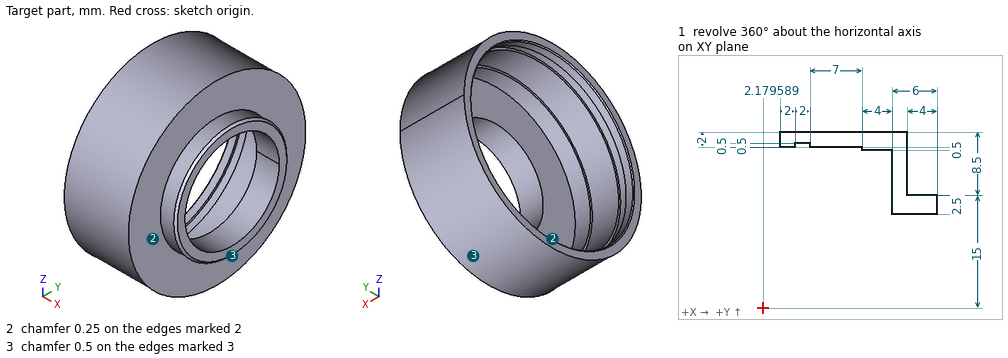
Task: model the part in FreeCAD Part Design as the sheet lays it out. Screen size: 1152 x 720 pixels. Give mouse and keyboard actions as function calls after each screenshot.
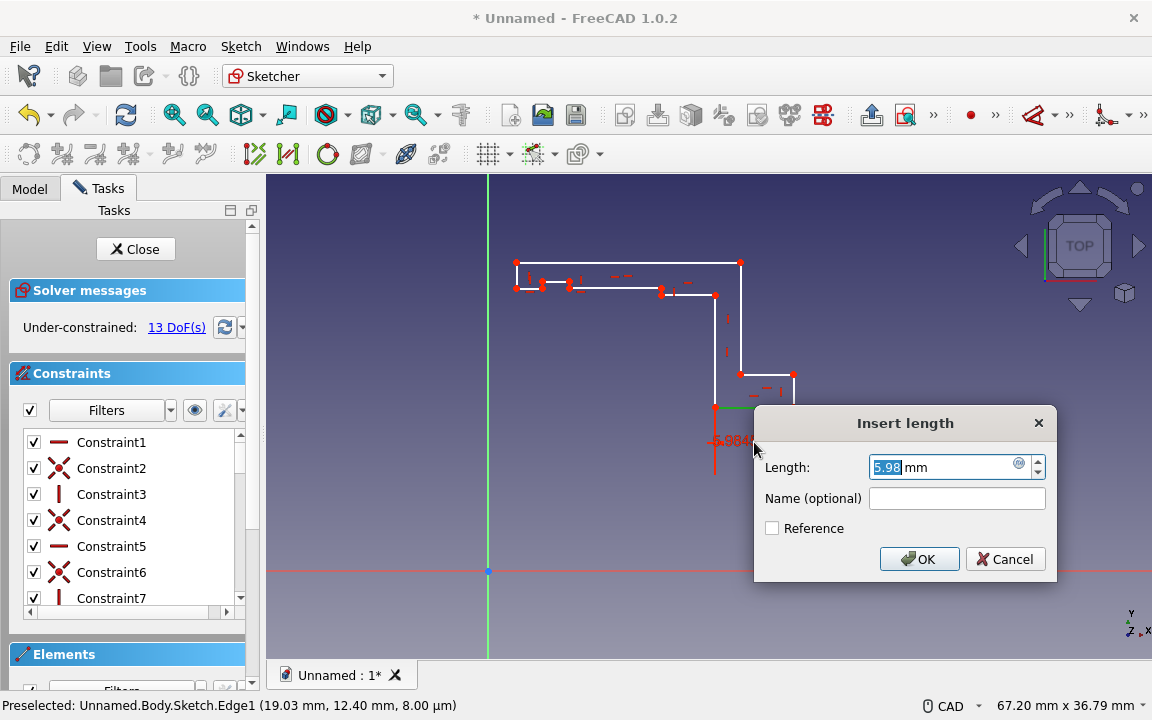
text(6)
key(Return)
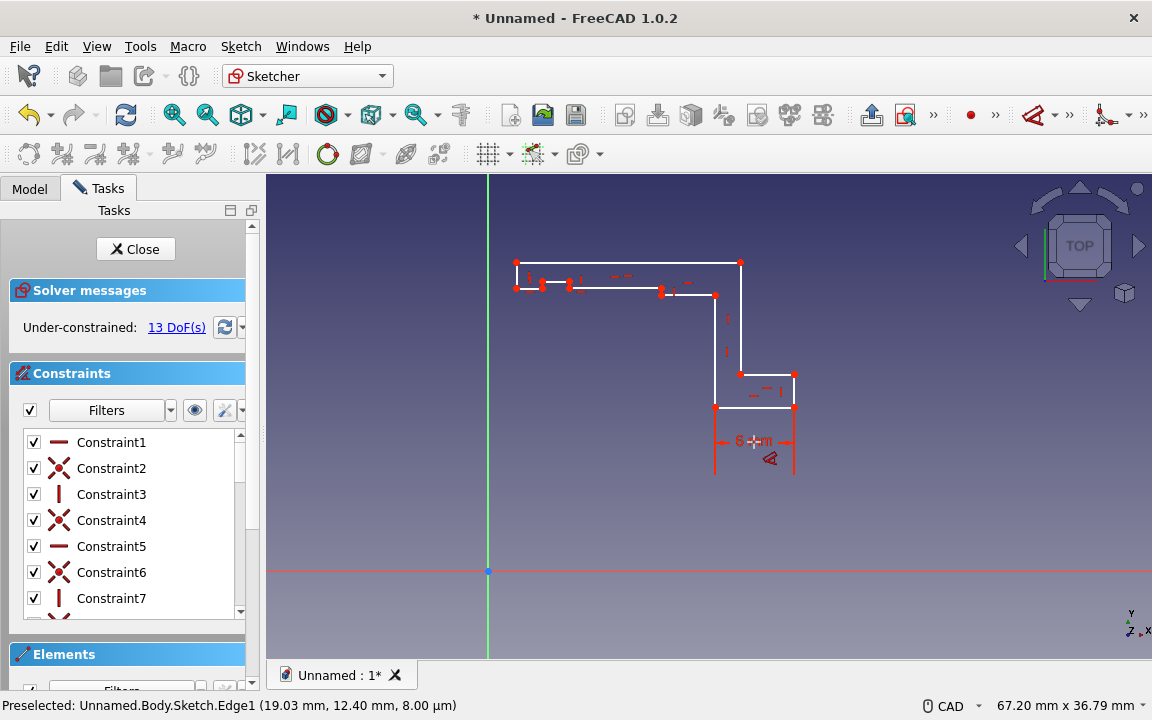
click(778, 375)
click(768, 341)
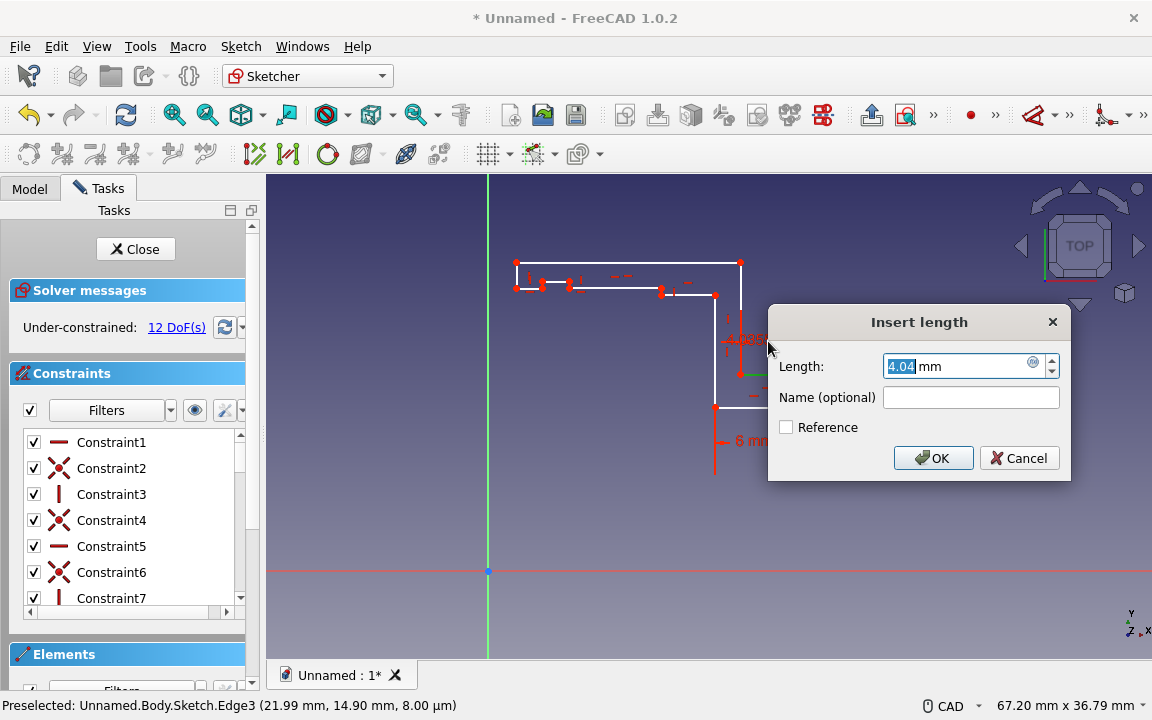
text(4)
key(Return)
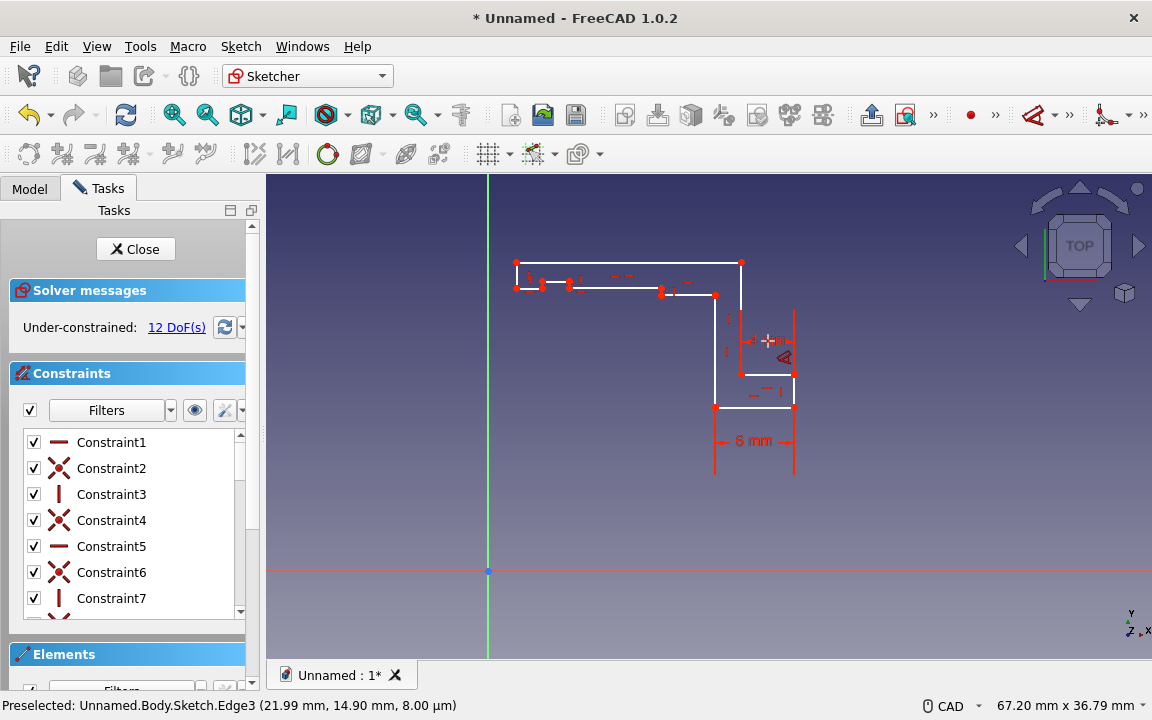
scroll(517, 273, up, 3)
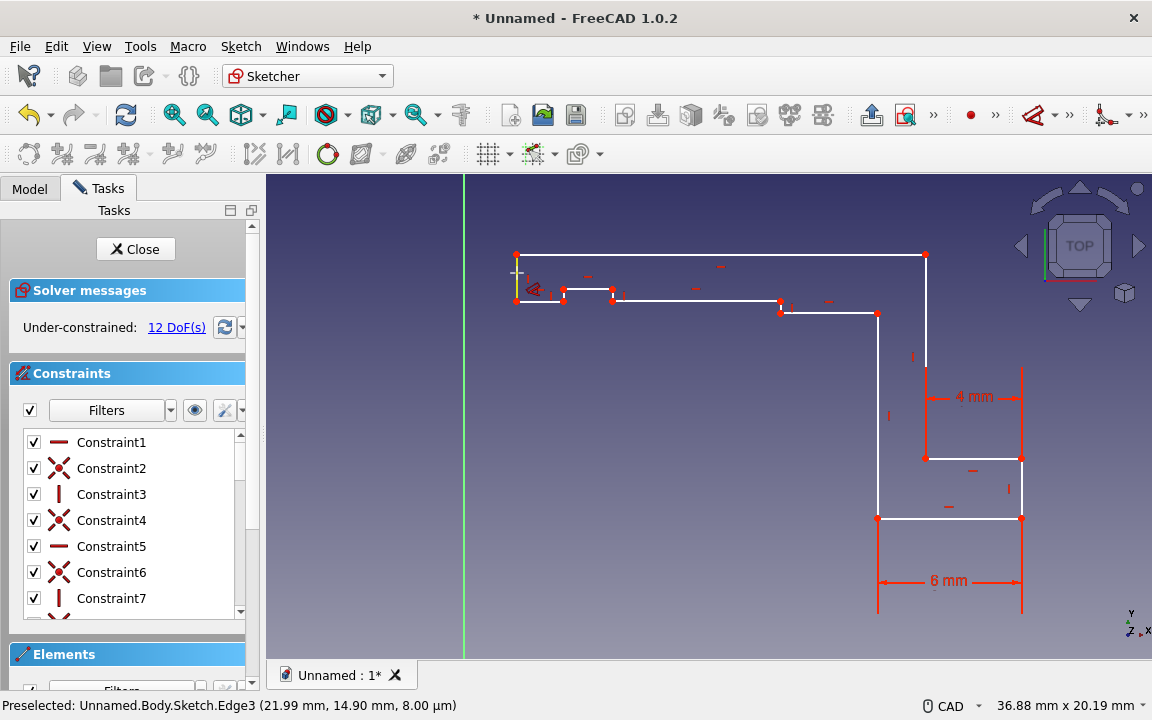
click(517, 274)
click(483, 278)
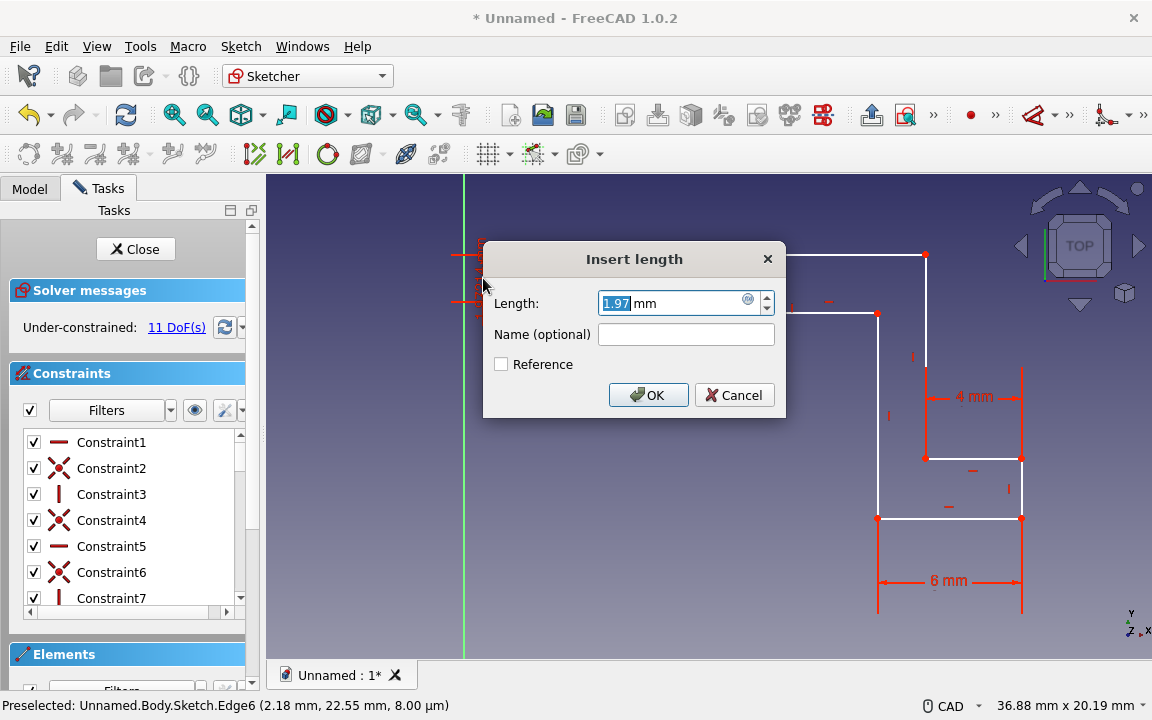
text(2)
key(Return)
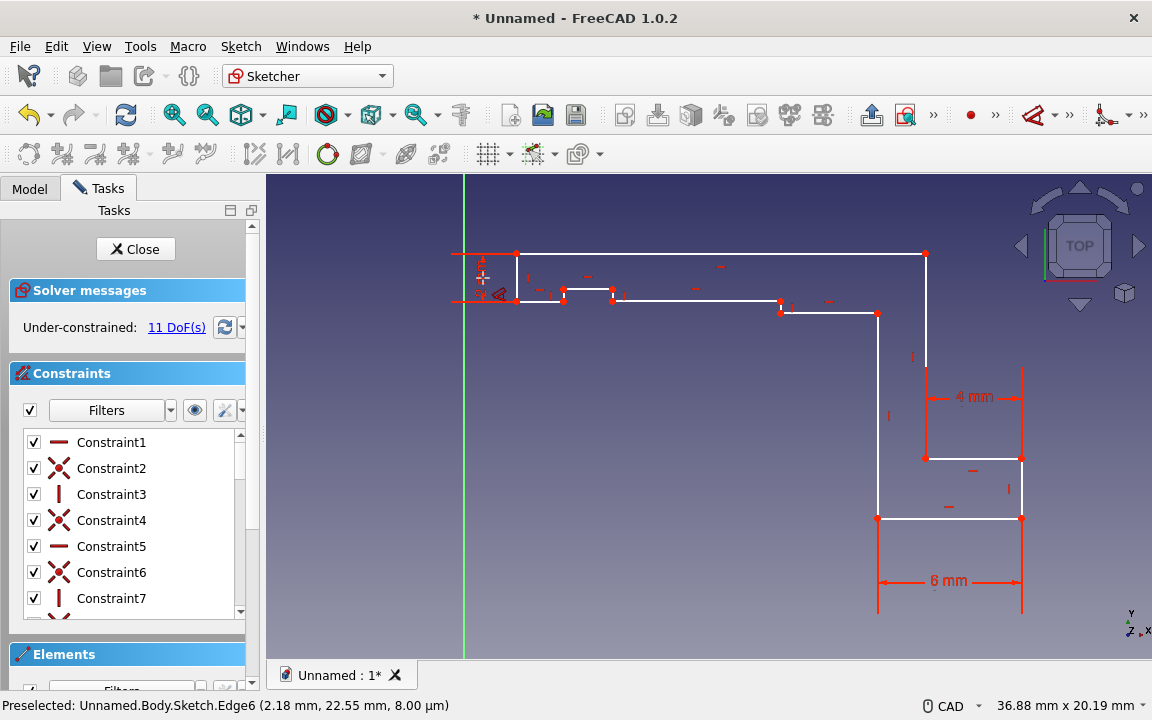
click(531, 302)
click(557, 268)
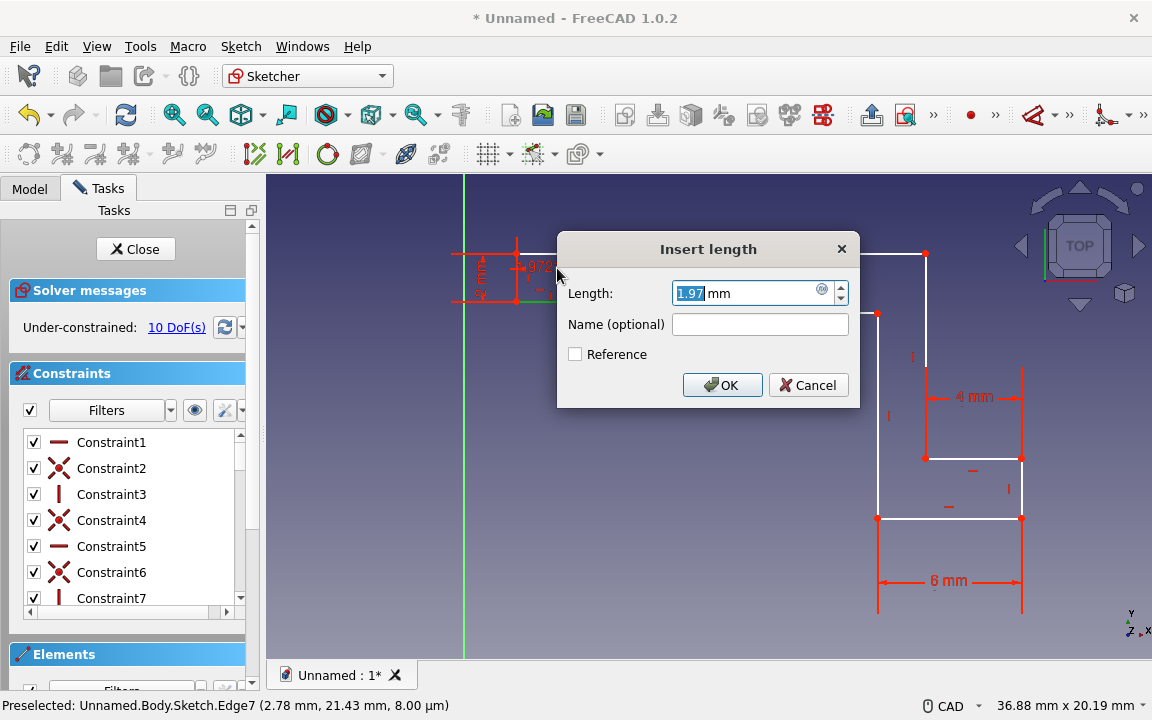
text(2)
key(Return)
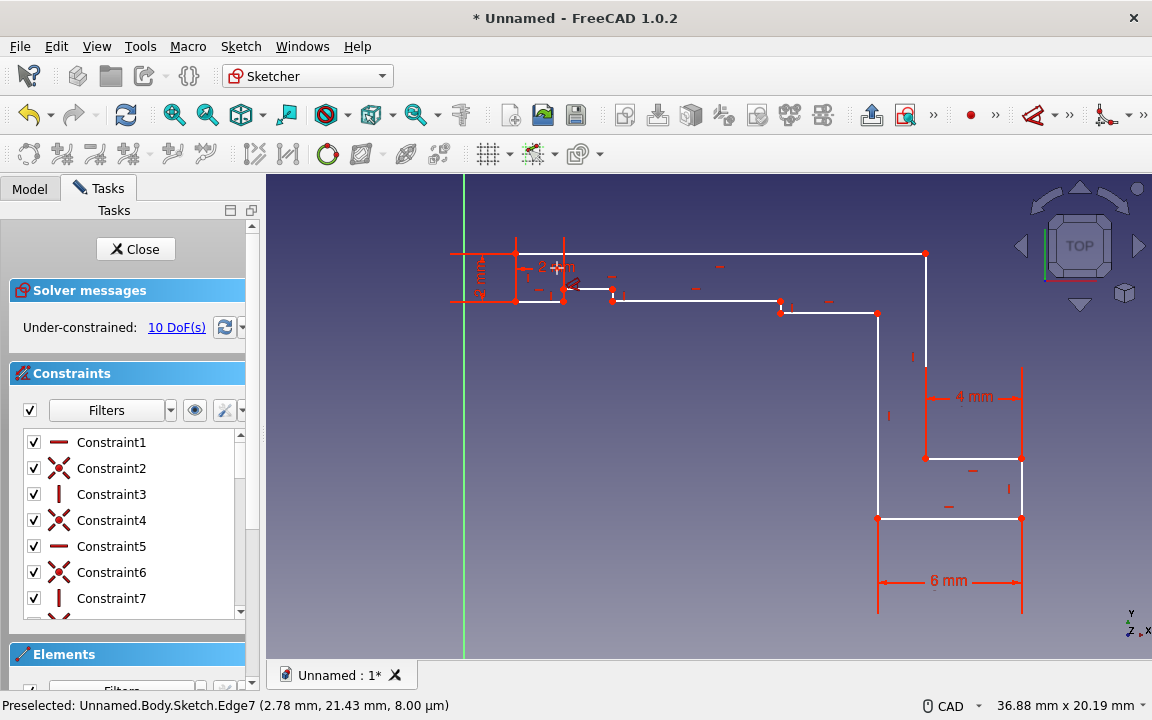
click(579, 289)
click(588, 323)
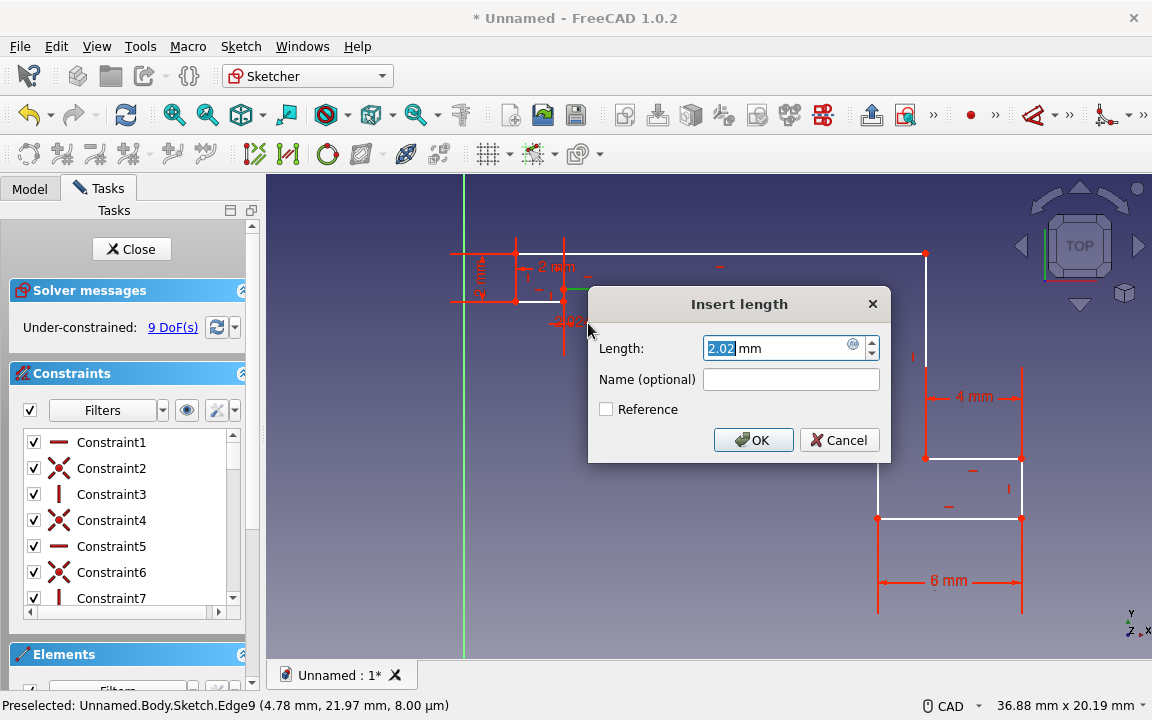
text(2)
key(Return)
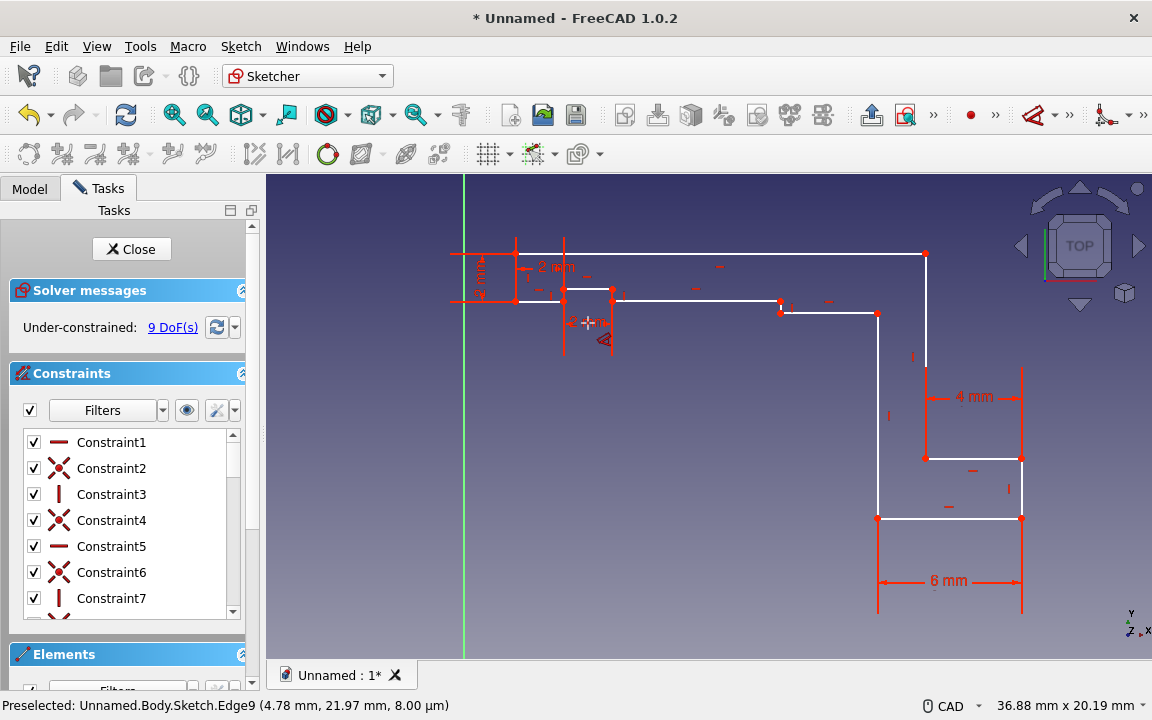
click(663, 301)
click(696, 267)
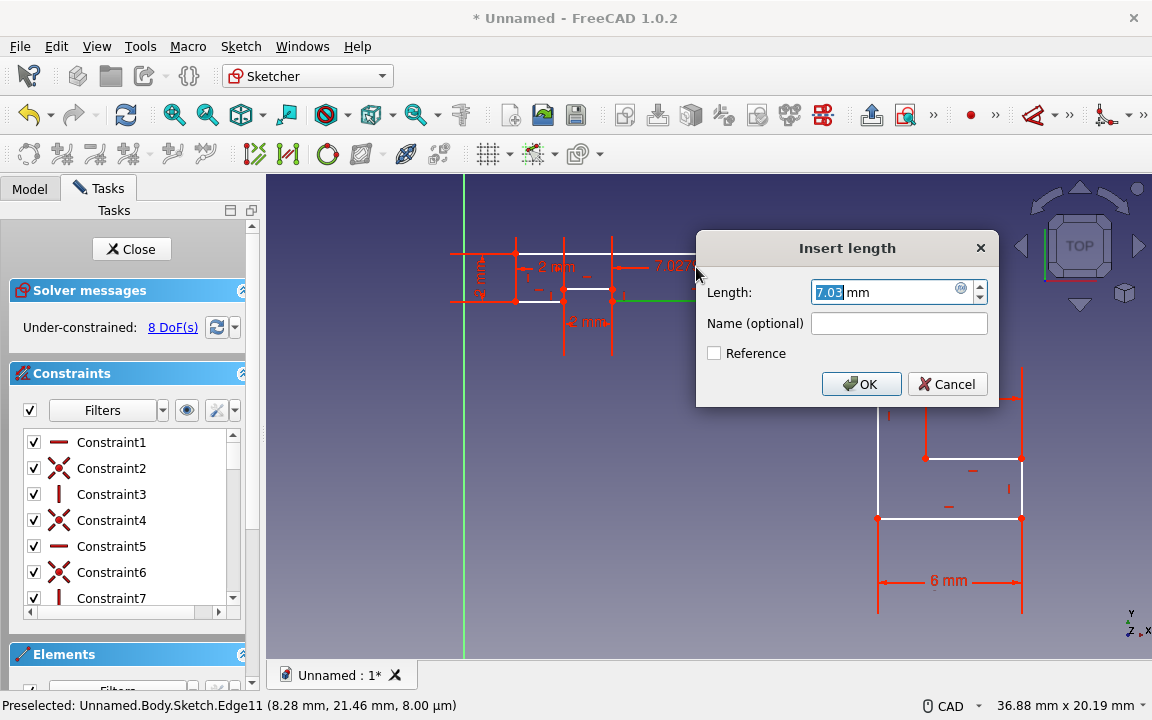
text(7)
key(Return)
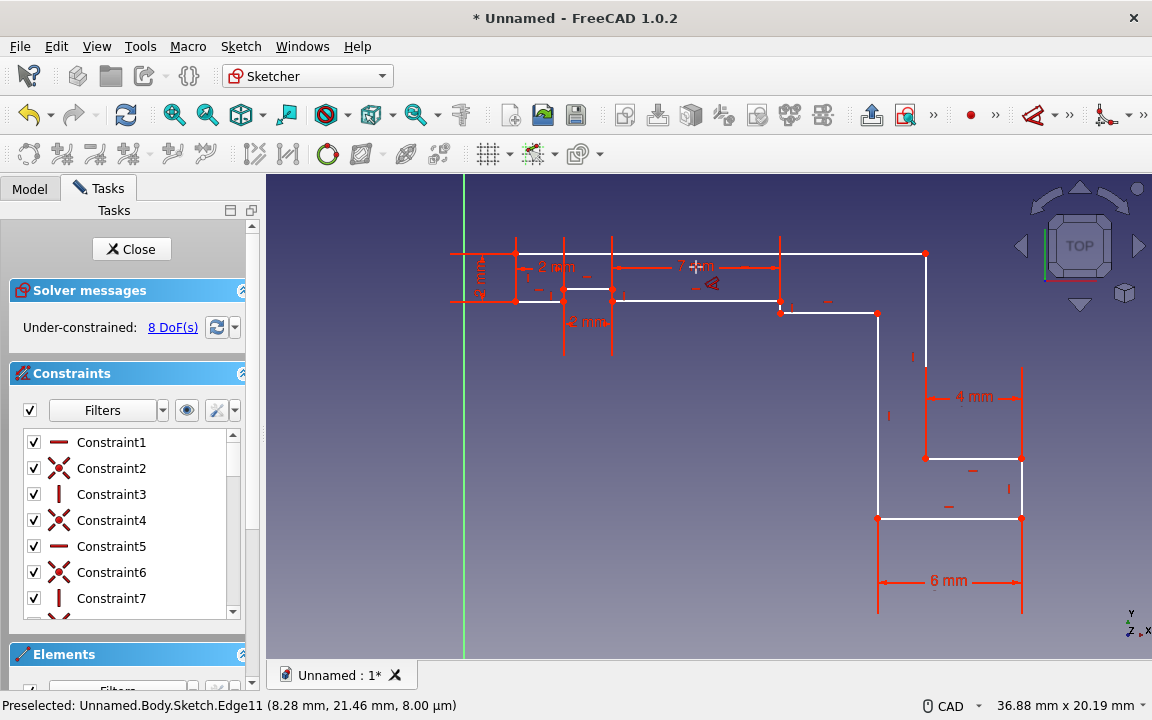
click(809, 313)
click(829, 279)